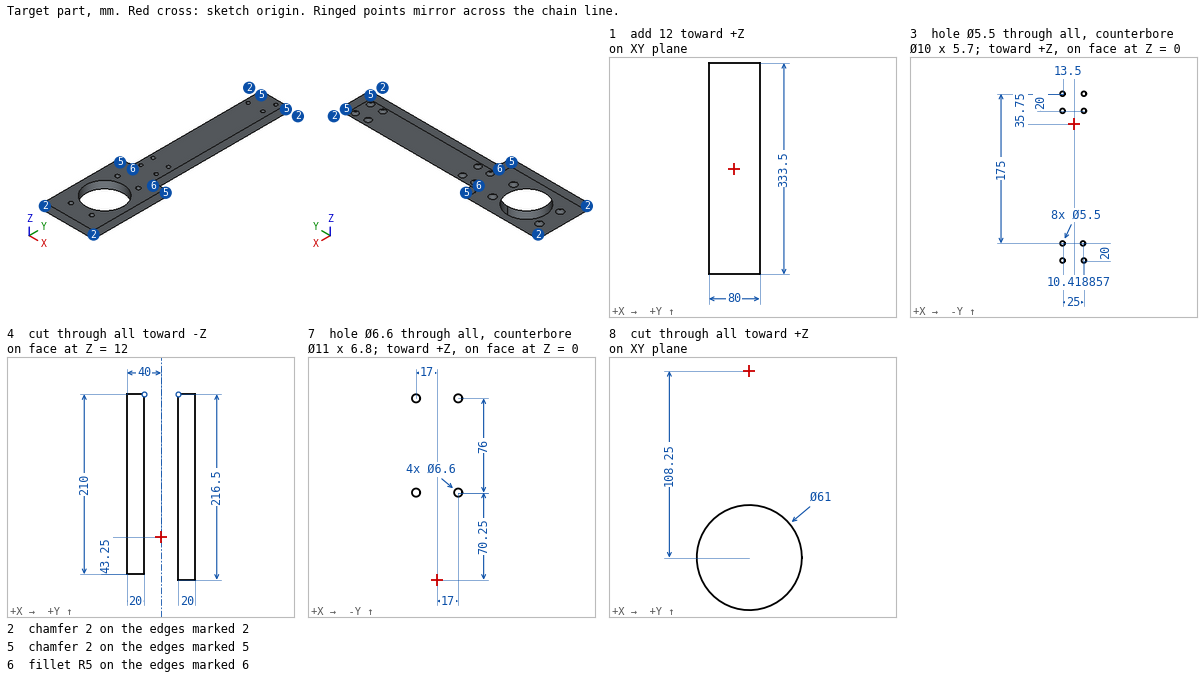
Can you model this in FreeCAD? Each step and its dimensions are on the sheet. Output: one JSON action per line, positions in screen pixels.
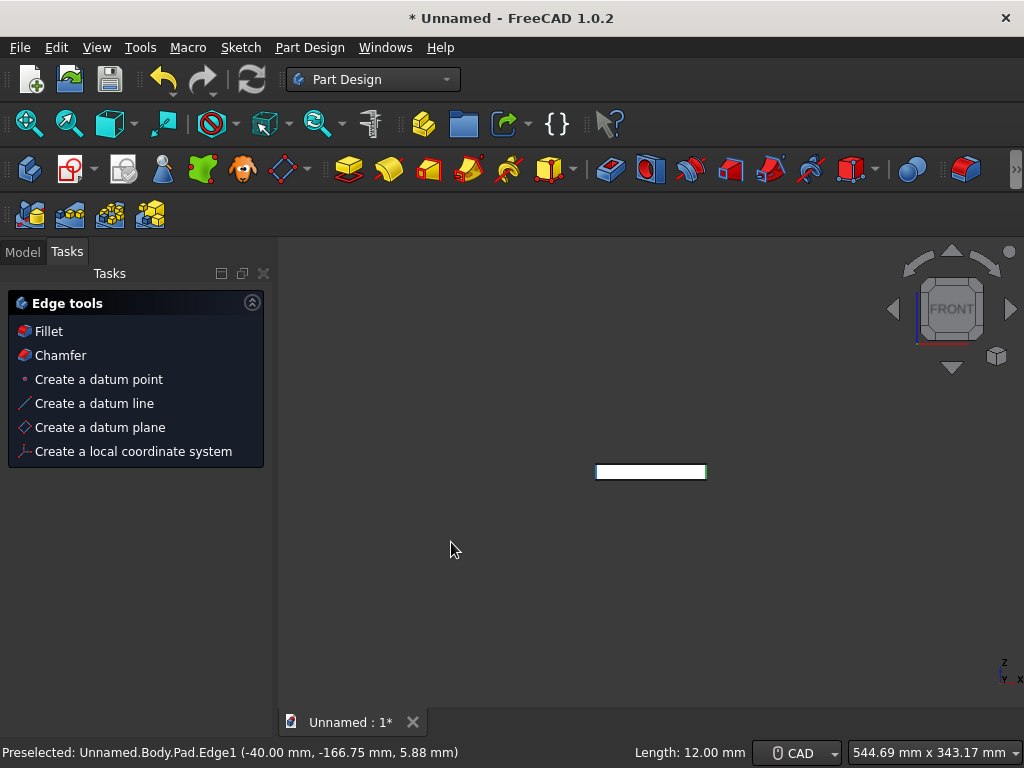
{"action": "left_click", "coordinate": [596, 471], "text": "ctrl"}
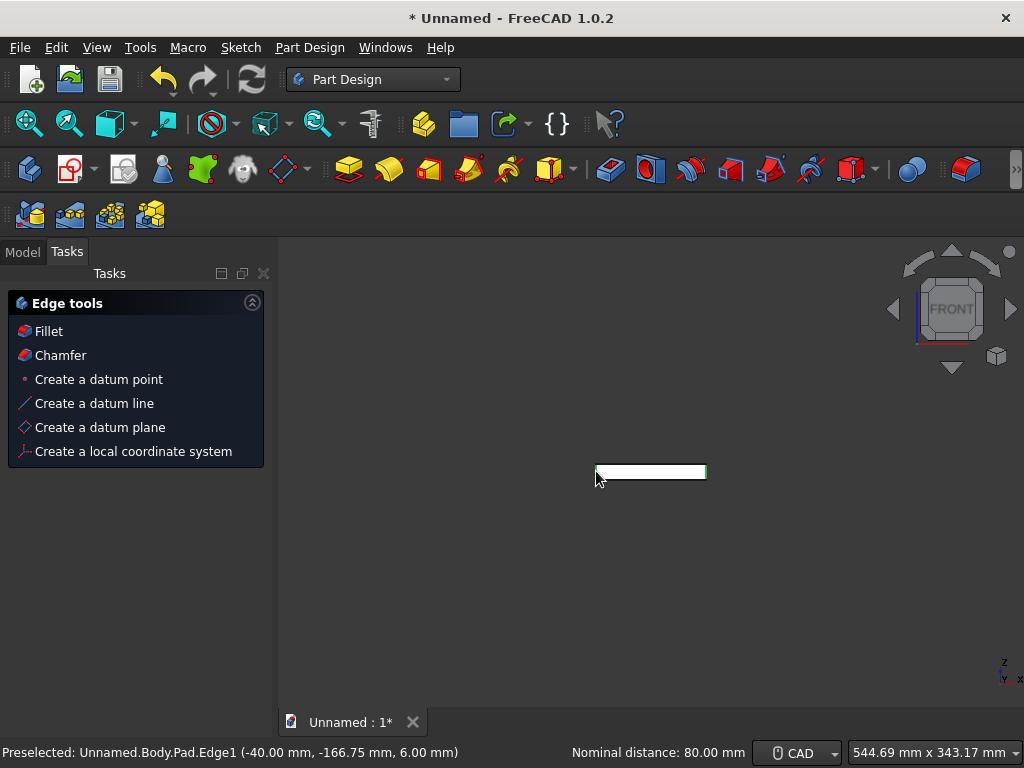
{"action": "scroll", "coordinate": [706, 471], "scroll_direction": "up", "scroll_amount": 5}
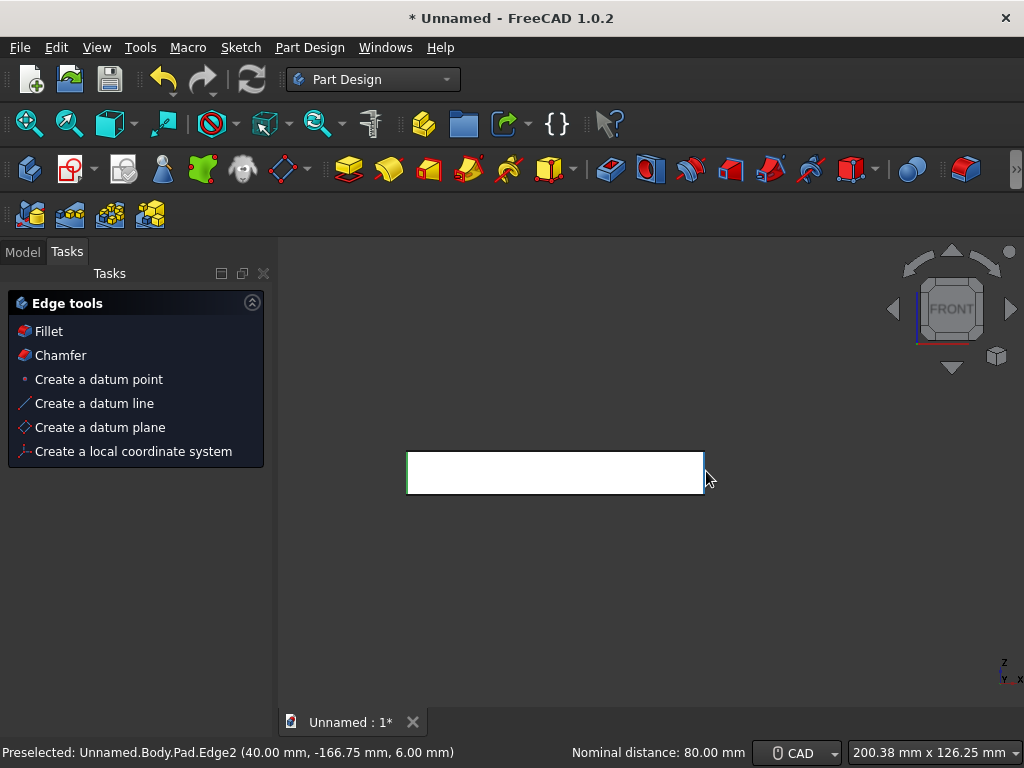
{"action": "key", "text": "v f"}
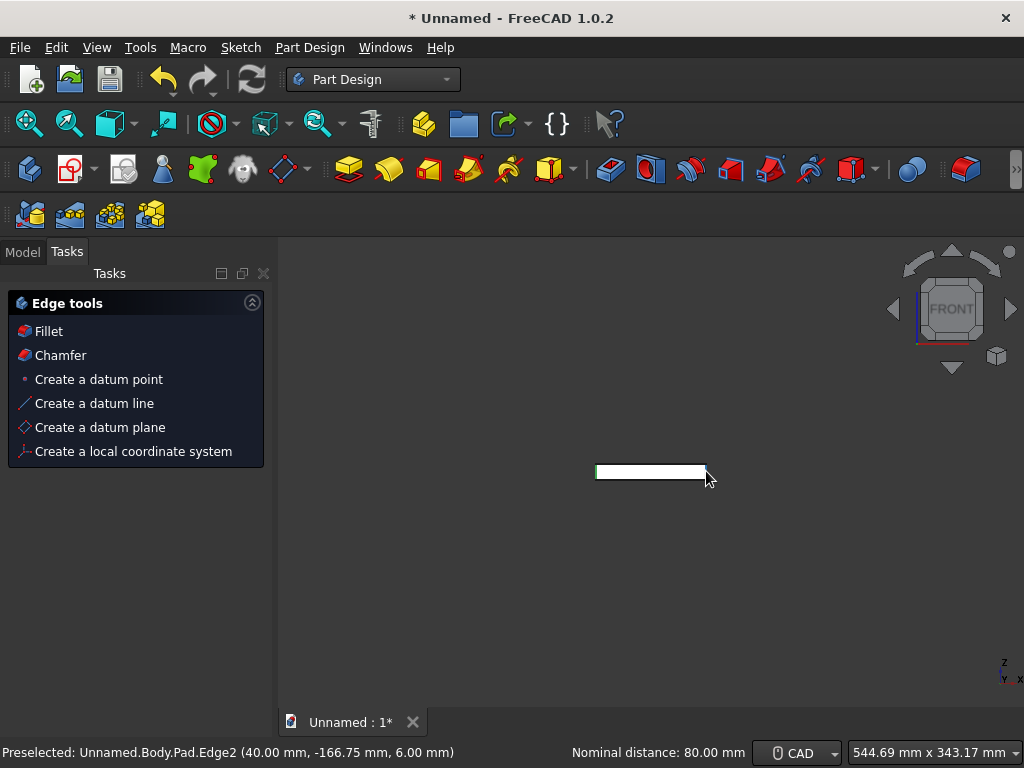
{"action": "key", "text": "3"}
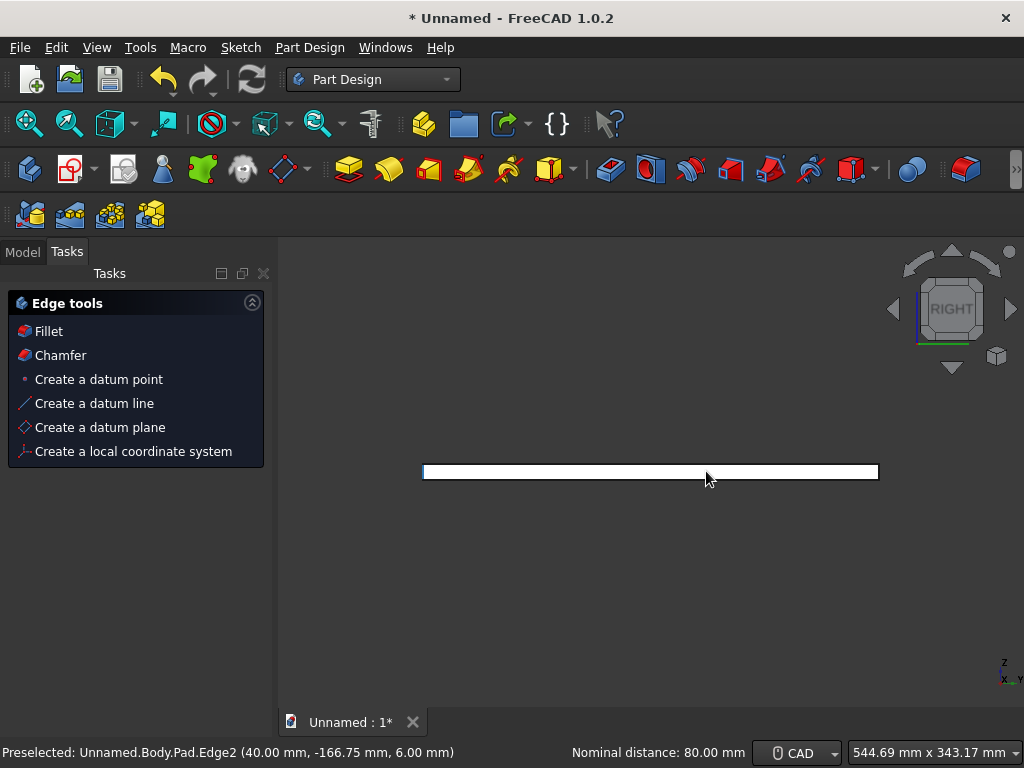
{"action": "left_click", "coordinate": [879, 471], "text": "ctrl"}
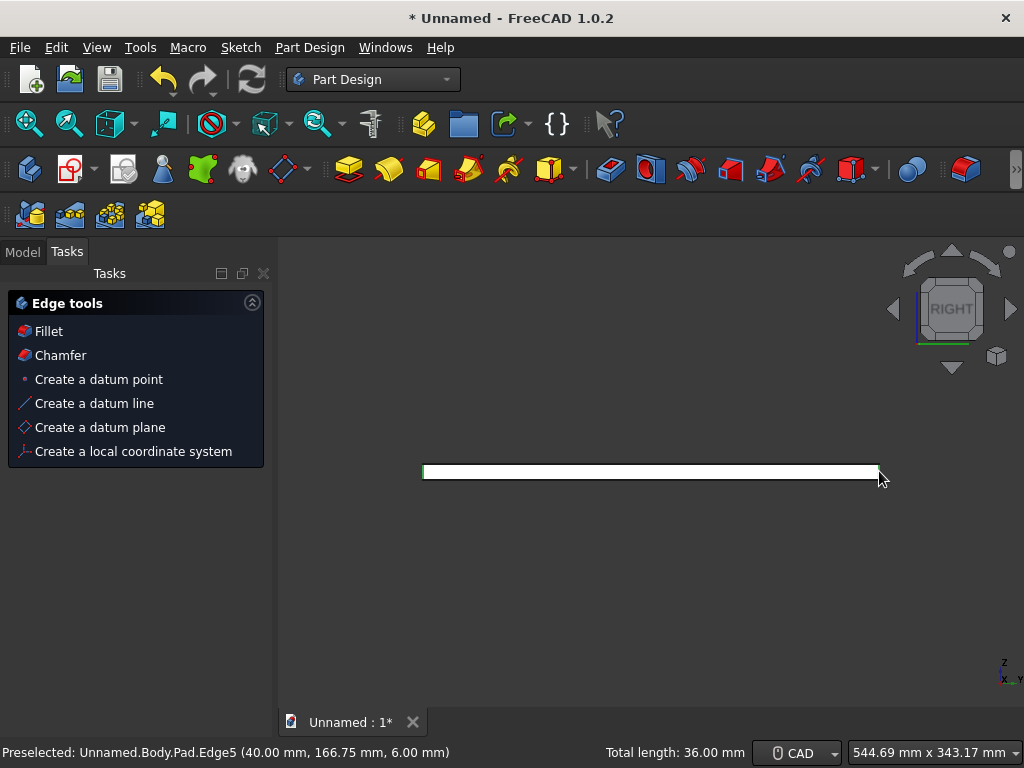
{"action": "key", "text": "5"}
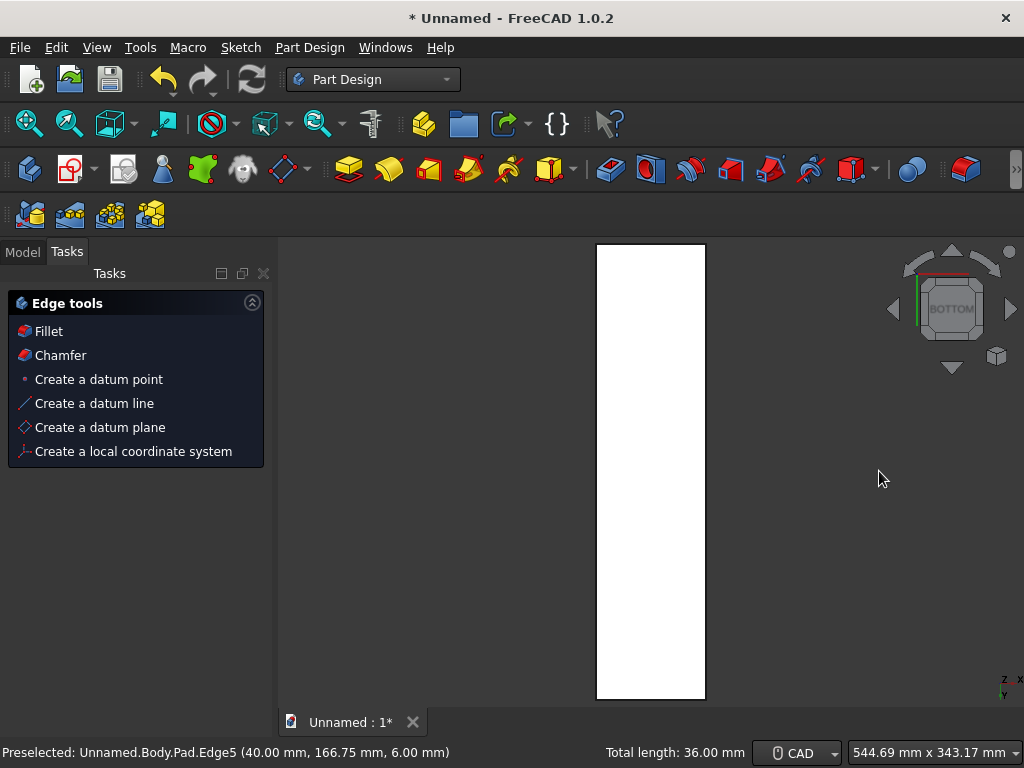
{"action": "key", "text": "4"}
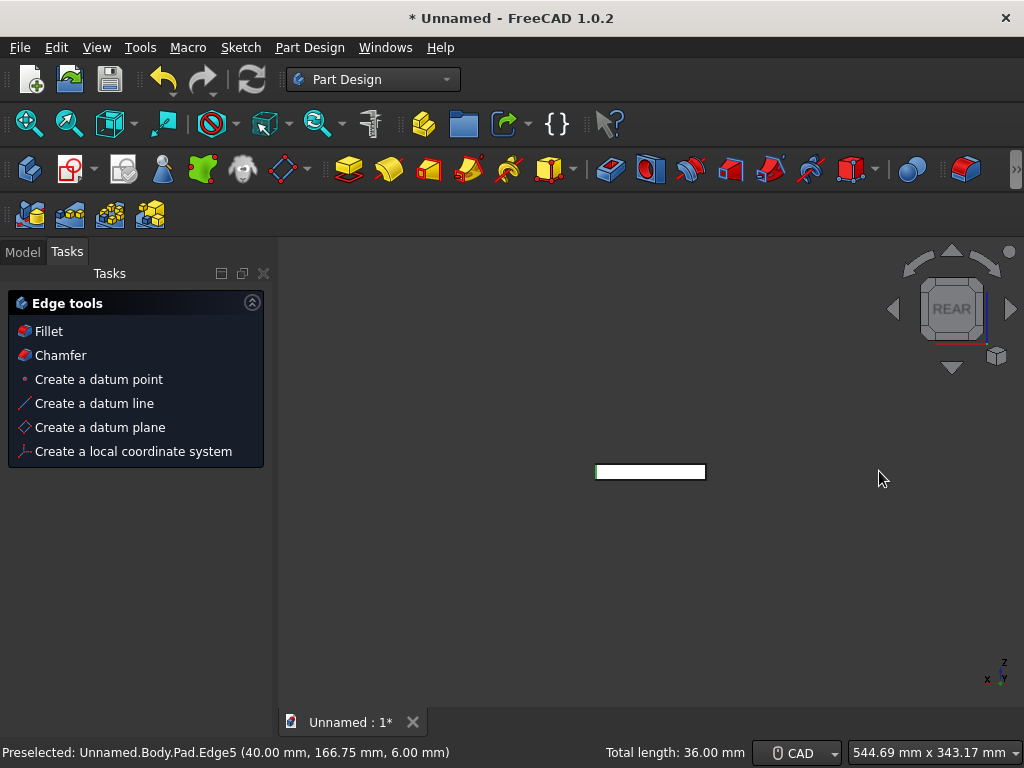
{"action": "left_click", "coordinate": [30, 124]}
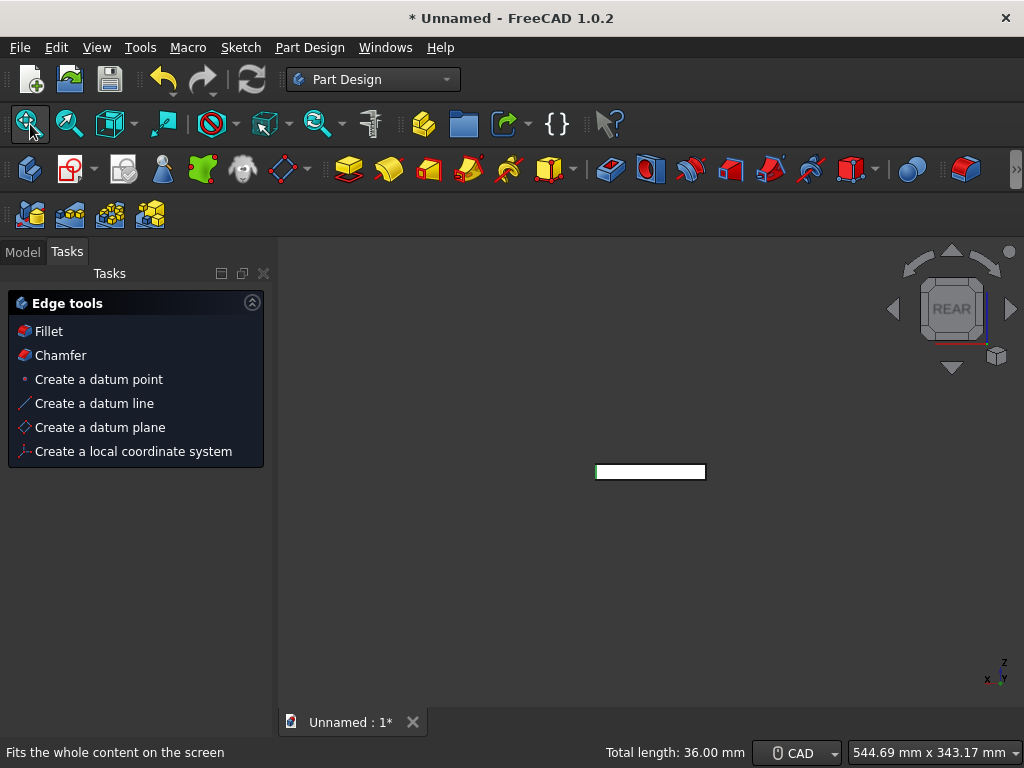
{"action": "left_click", "coordinate": [706, 471], "text": "ctrl"}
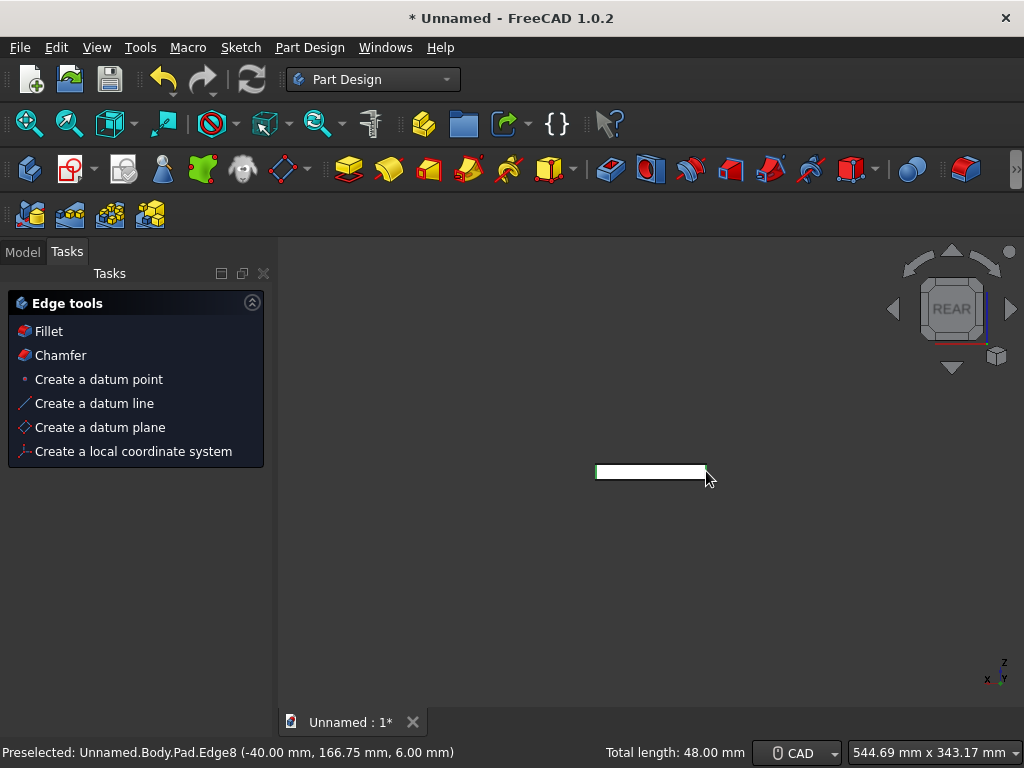
{"action": "left_click", "coordinate": [136, 355]}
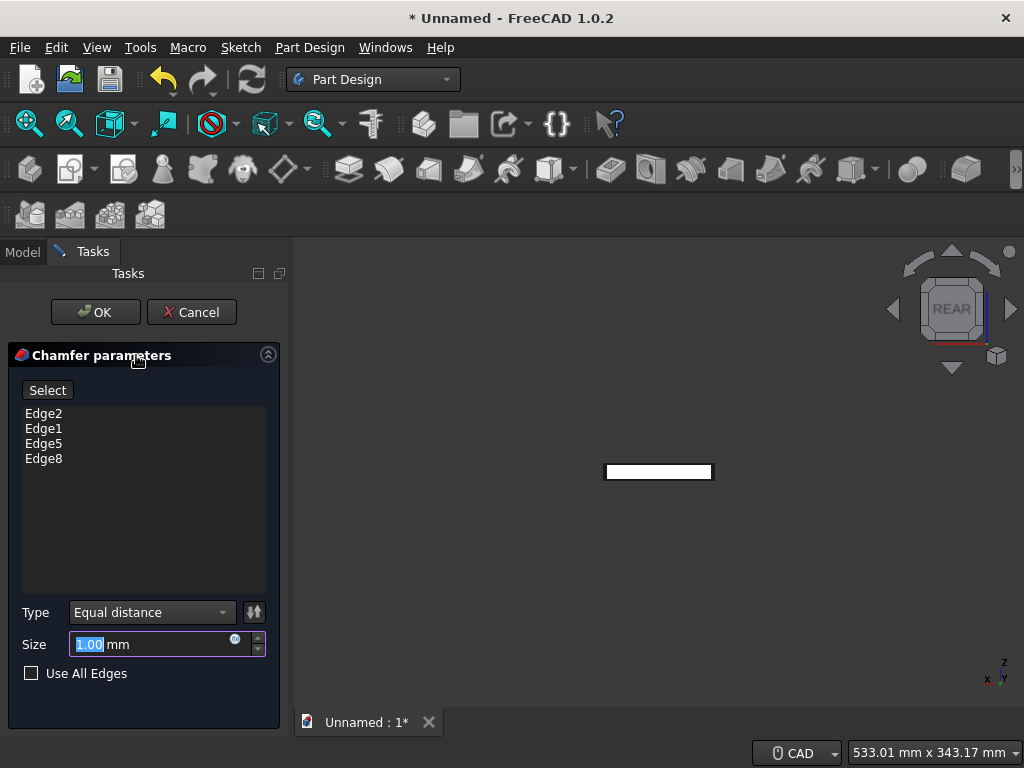
{"action": "type", "text": "2"}
{"action": "key", "text": "Tab"}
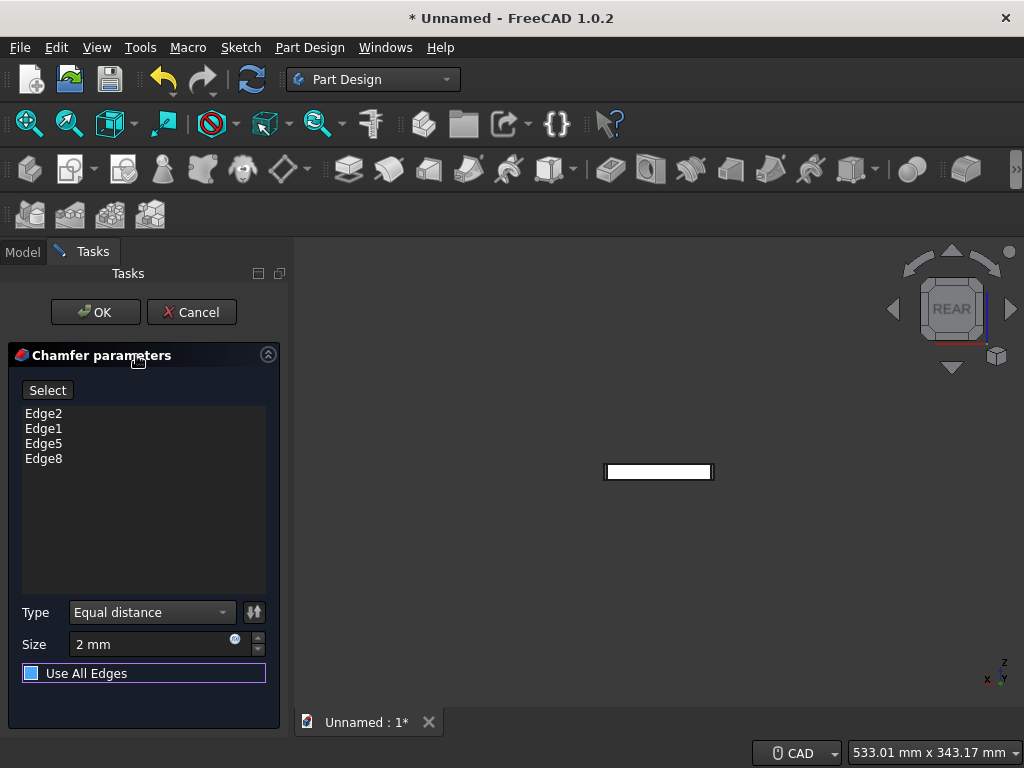
{"action": "left_click", "coordinate": [96, 312]}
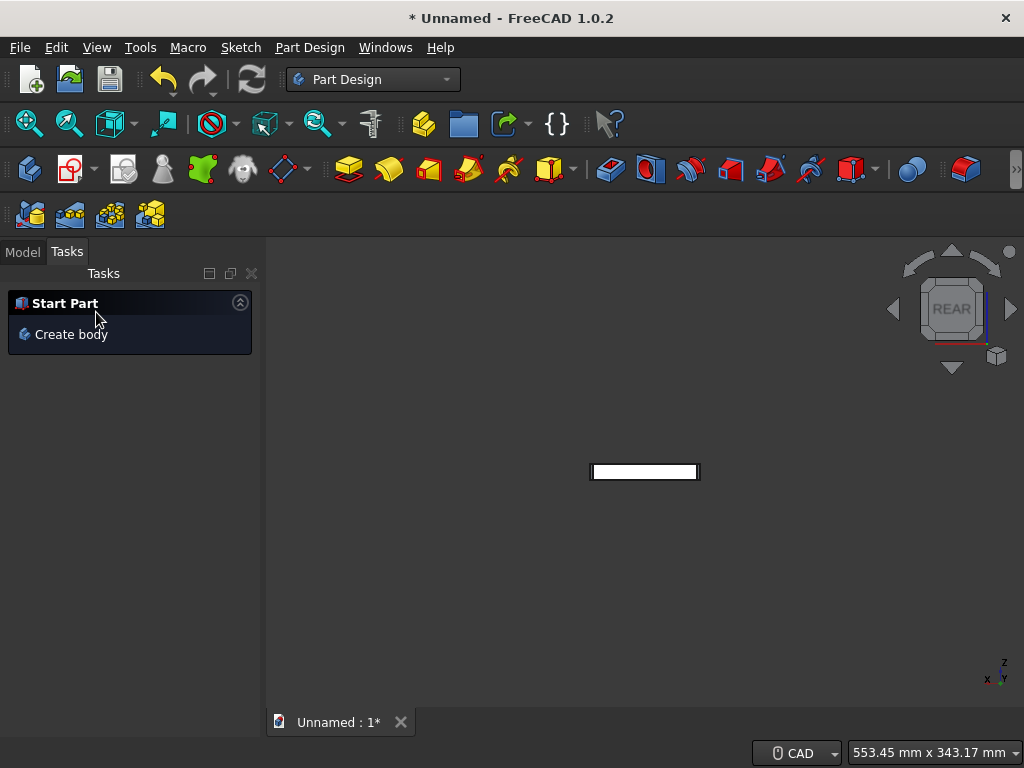
{"action": "key", "text": "v f"}